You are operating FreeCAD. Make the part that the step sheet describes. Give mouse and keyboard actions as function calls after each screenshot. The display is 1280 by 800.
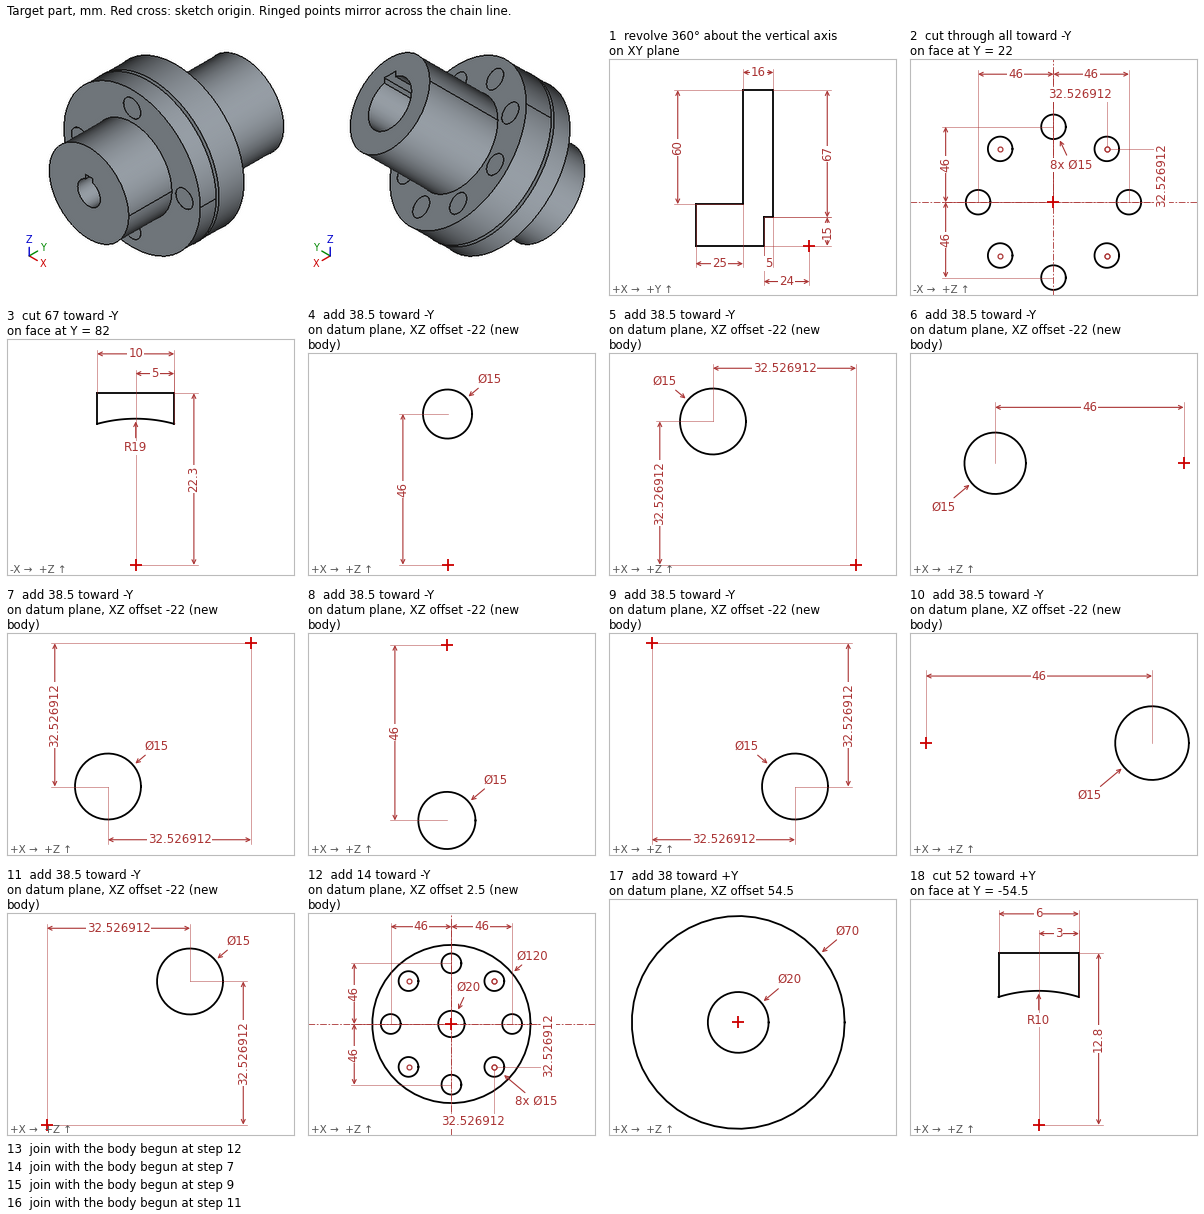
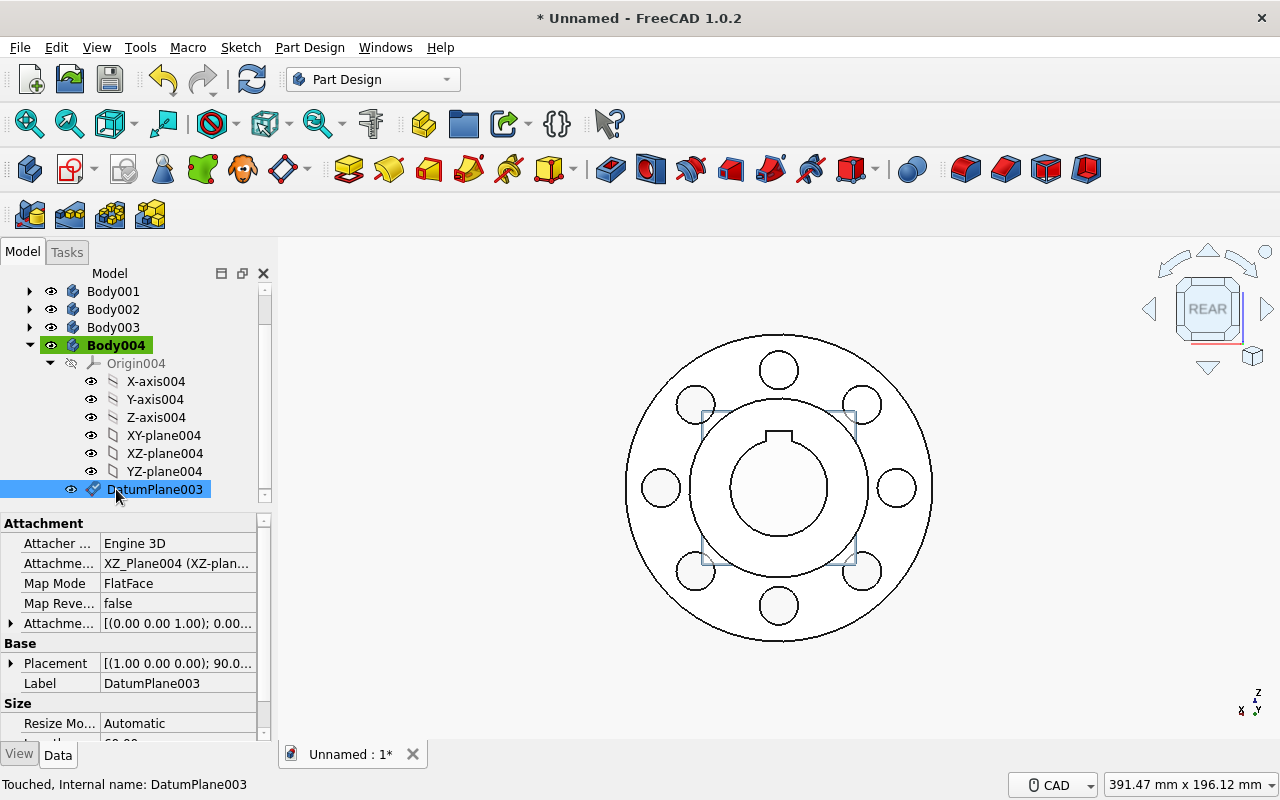
click(70, 170)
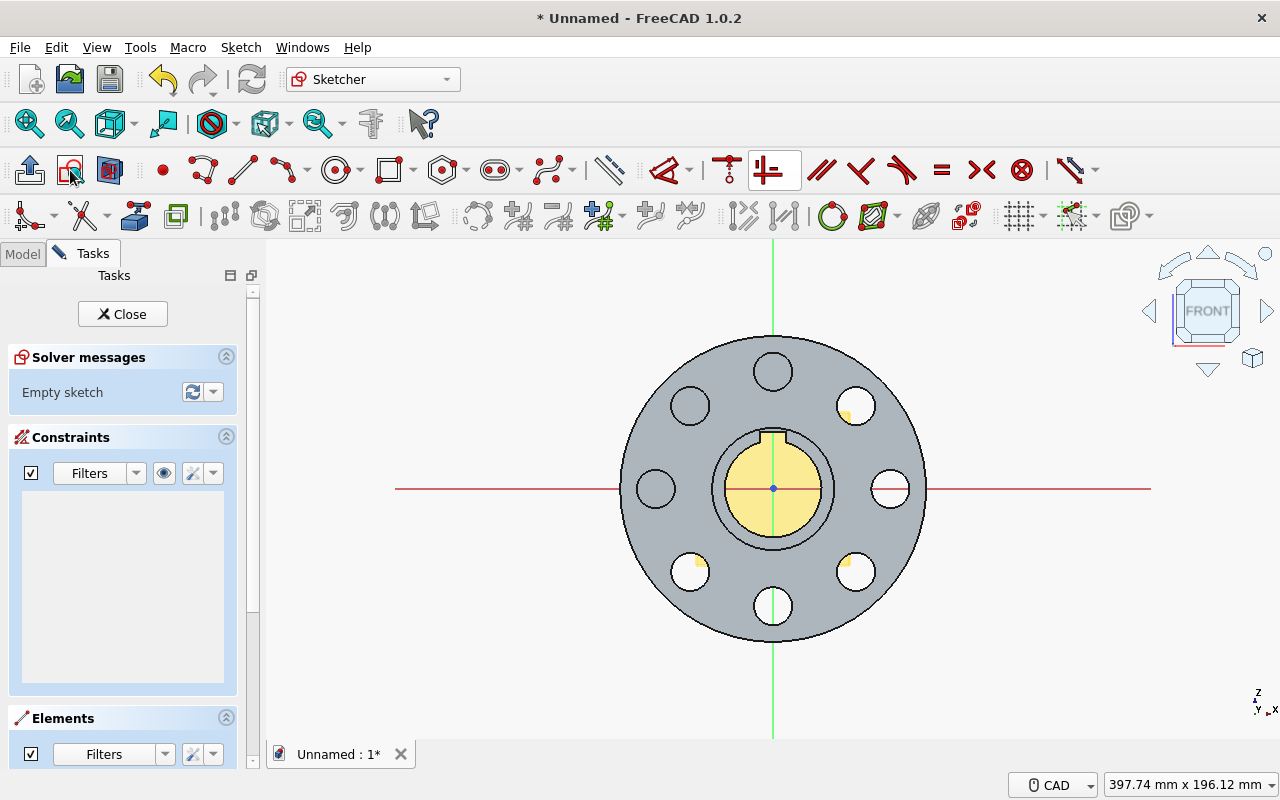
scroll(688, 582, up, 11)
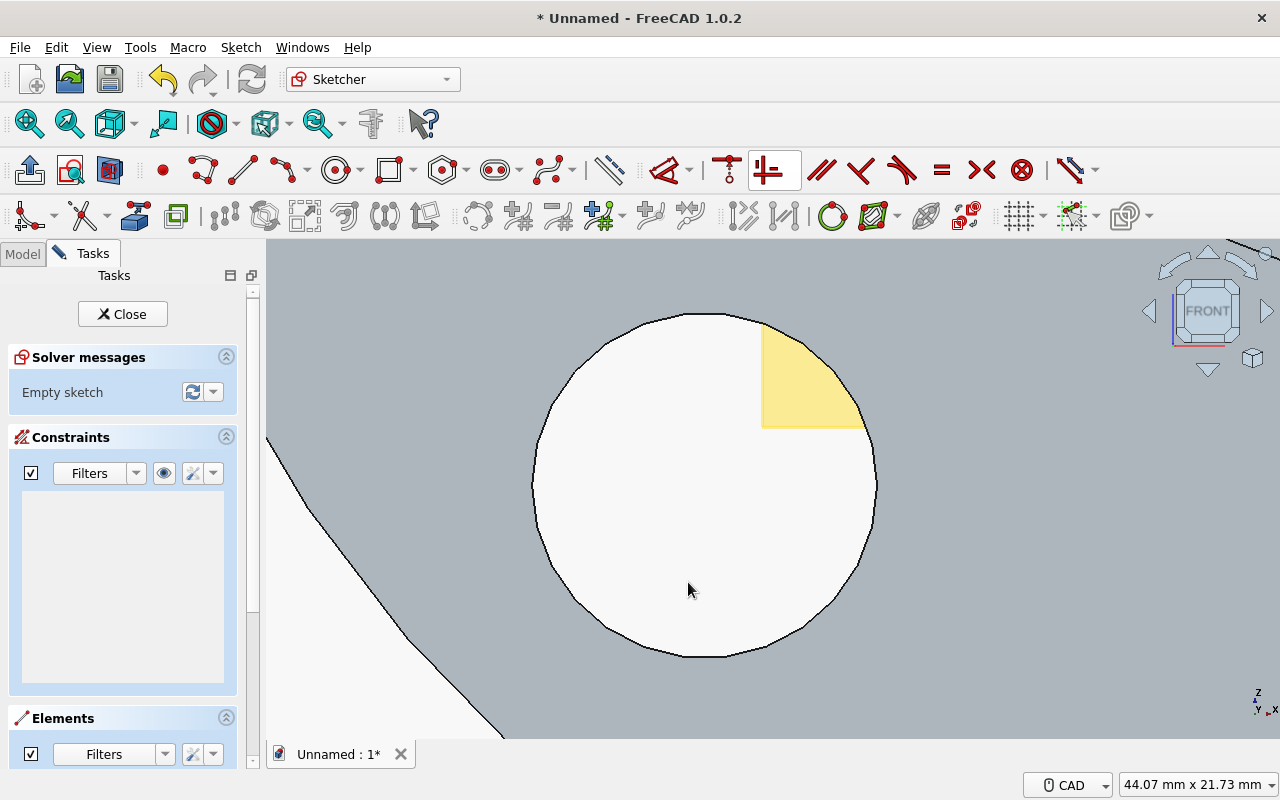
click(336, 170)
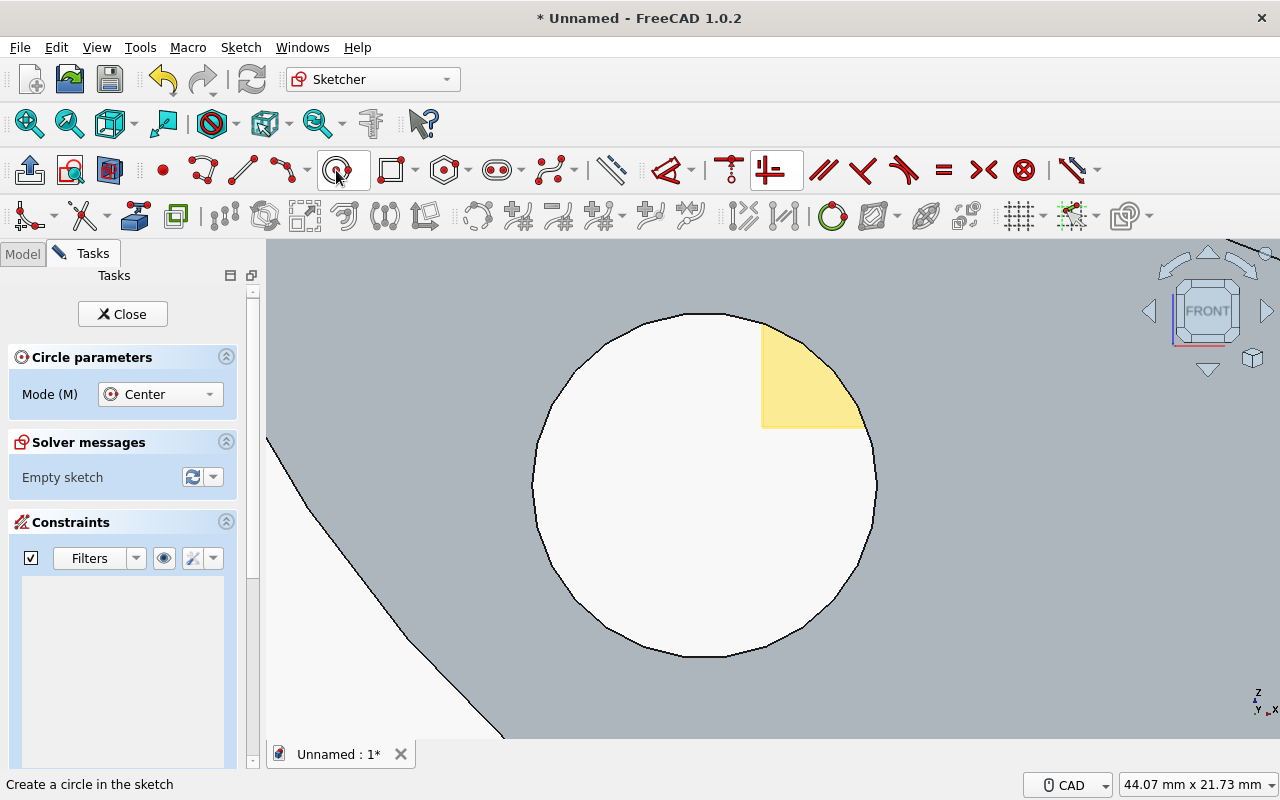
click(705, 486)
click(827, 364)
key(Escape)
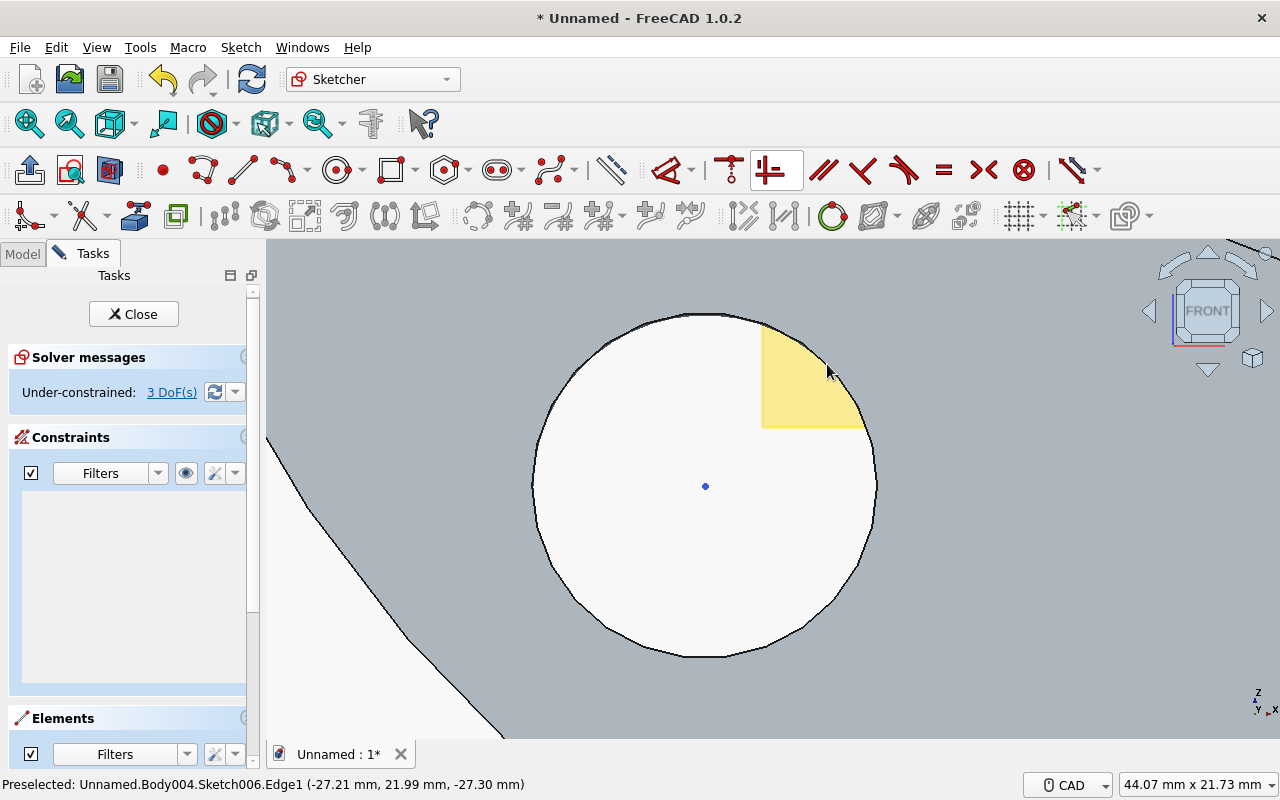
click(666, 170)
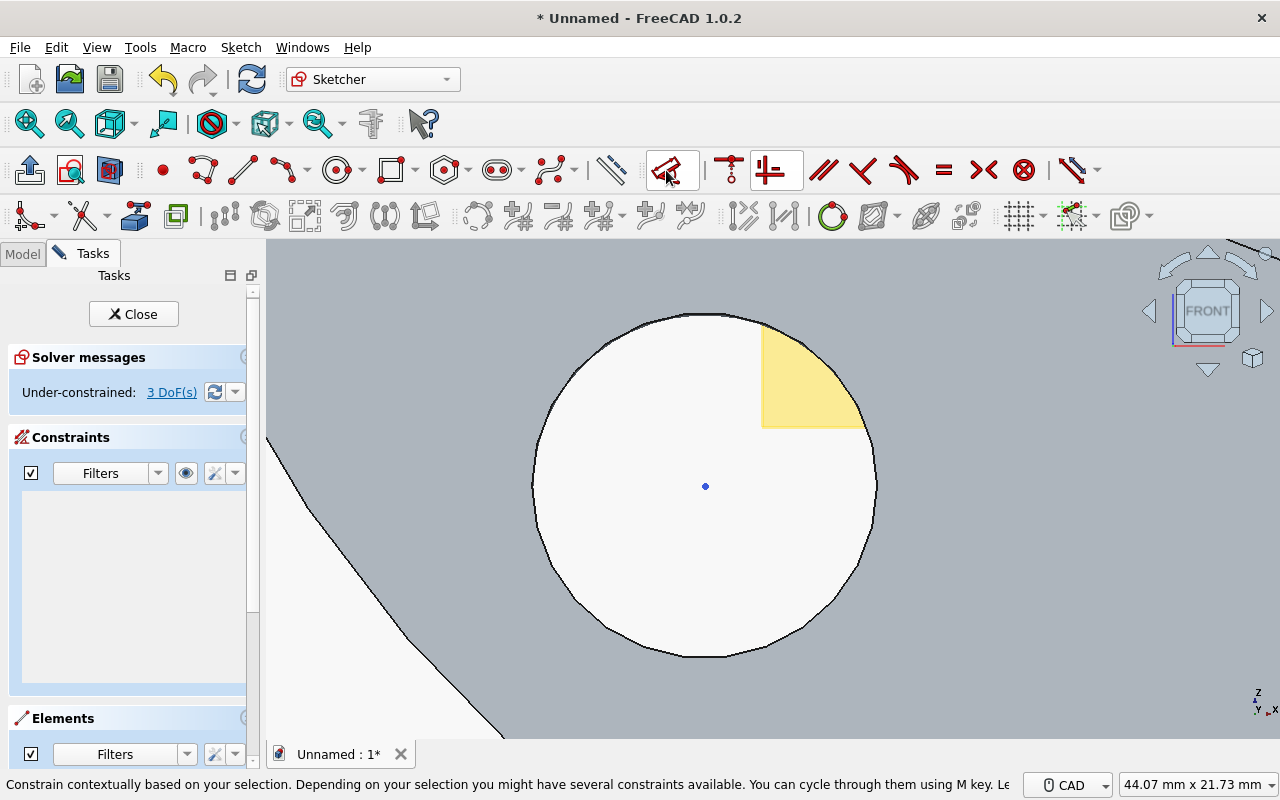
click(827, 365)
click(850, 342)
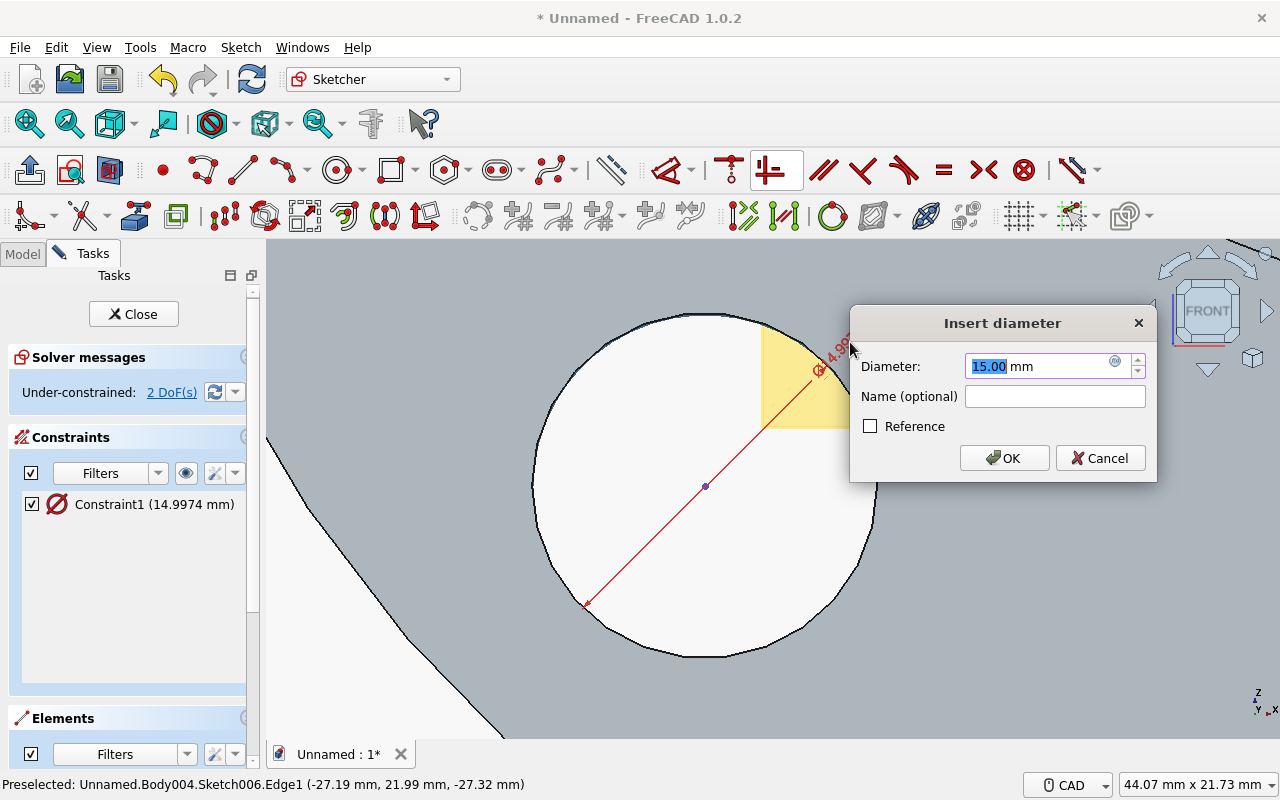
text(15)
key(Return)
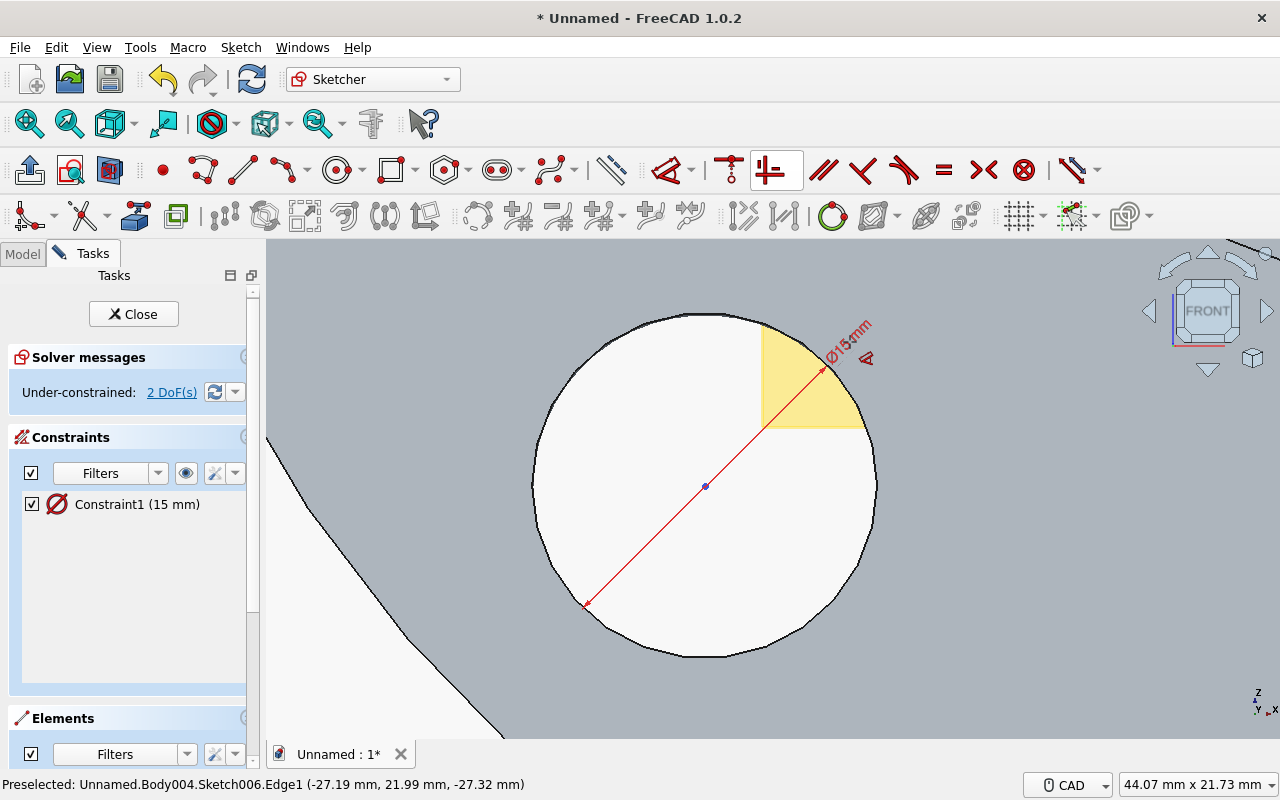
click(705, 487)
click(910, 521)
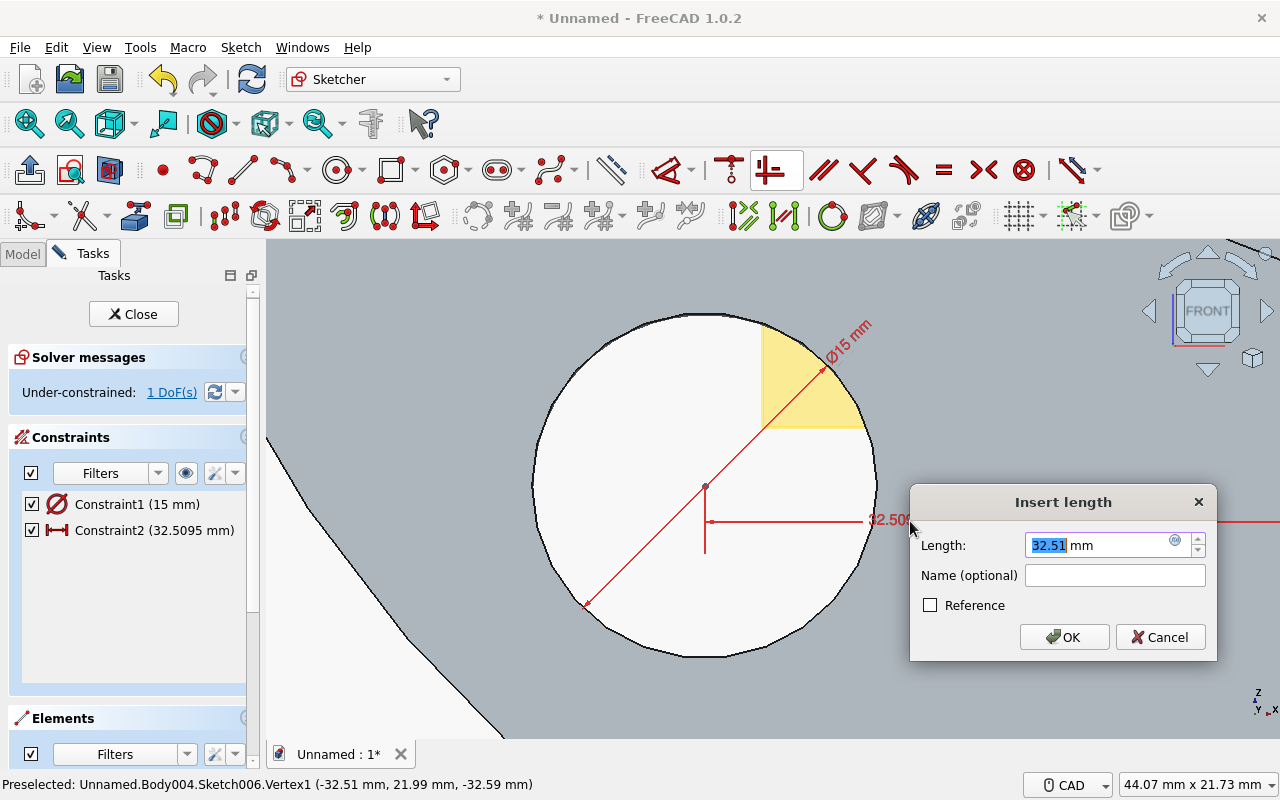
text(32.526912)
key(Return)